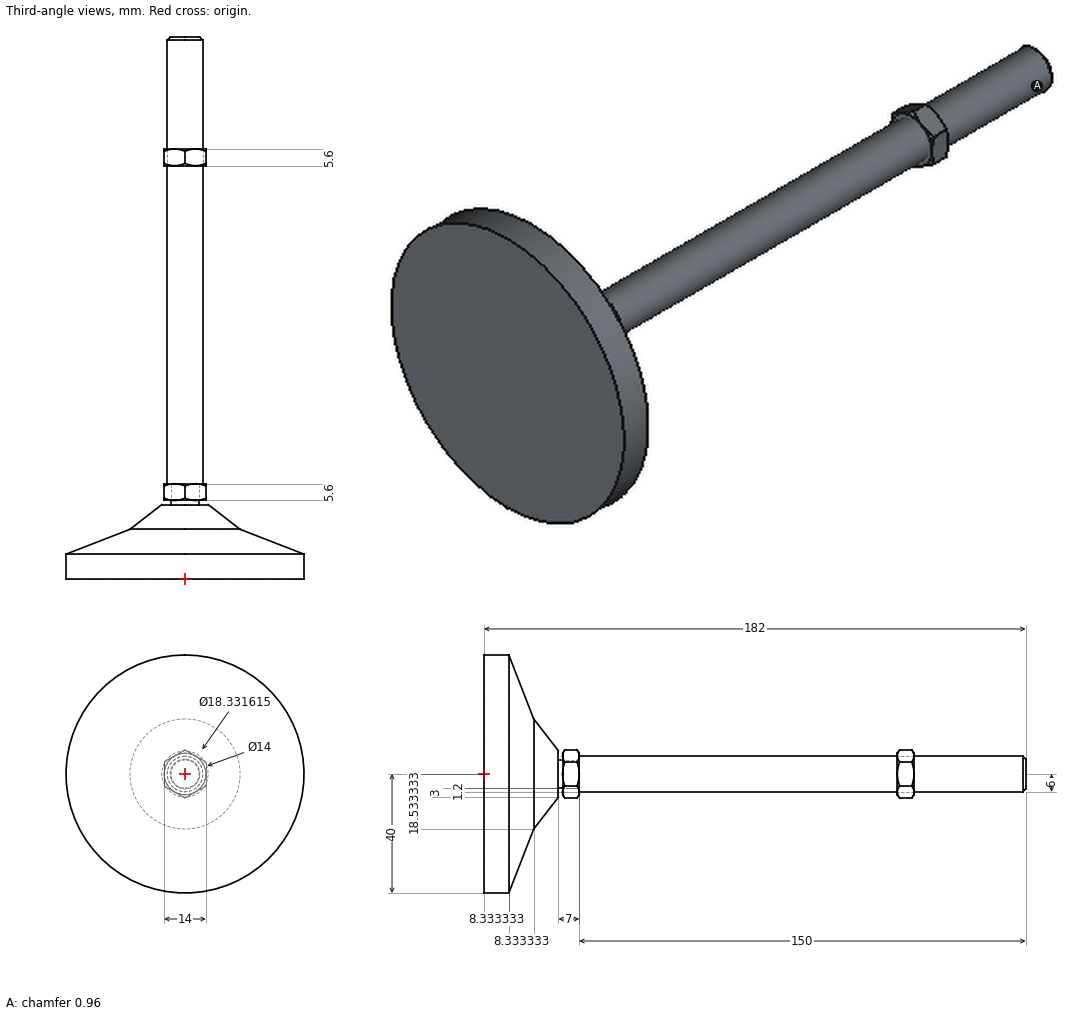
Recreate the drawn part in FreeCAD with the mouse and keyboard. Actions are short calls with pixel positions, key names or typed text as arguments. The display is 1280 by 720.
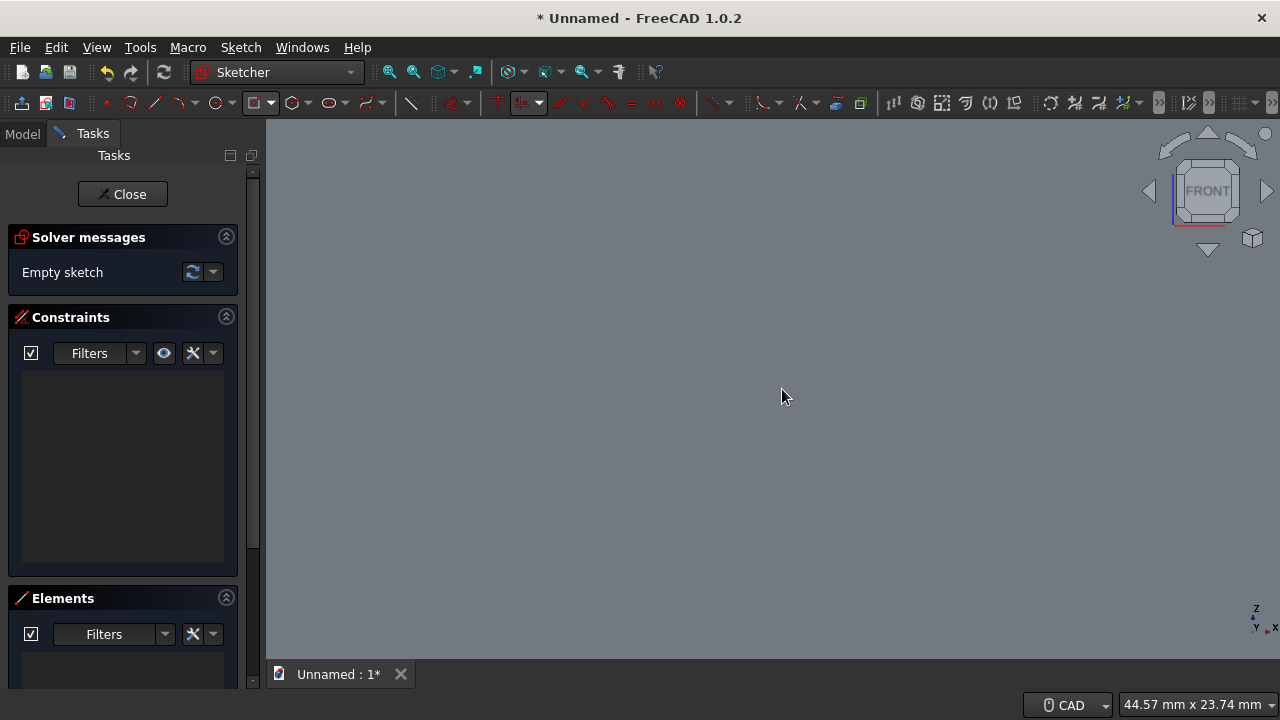
click(292, 104)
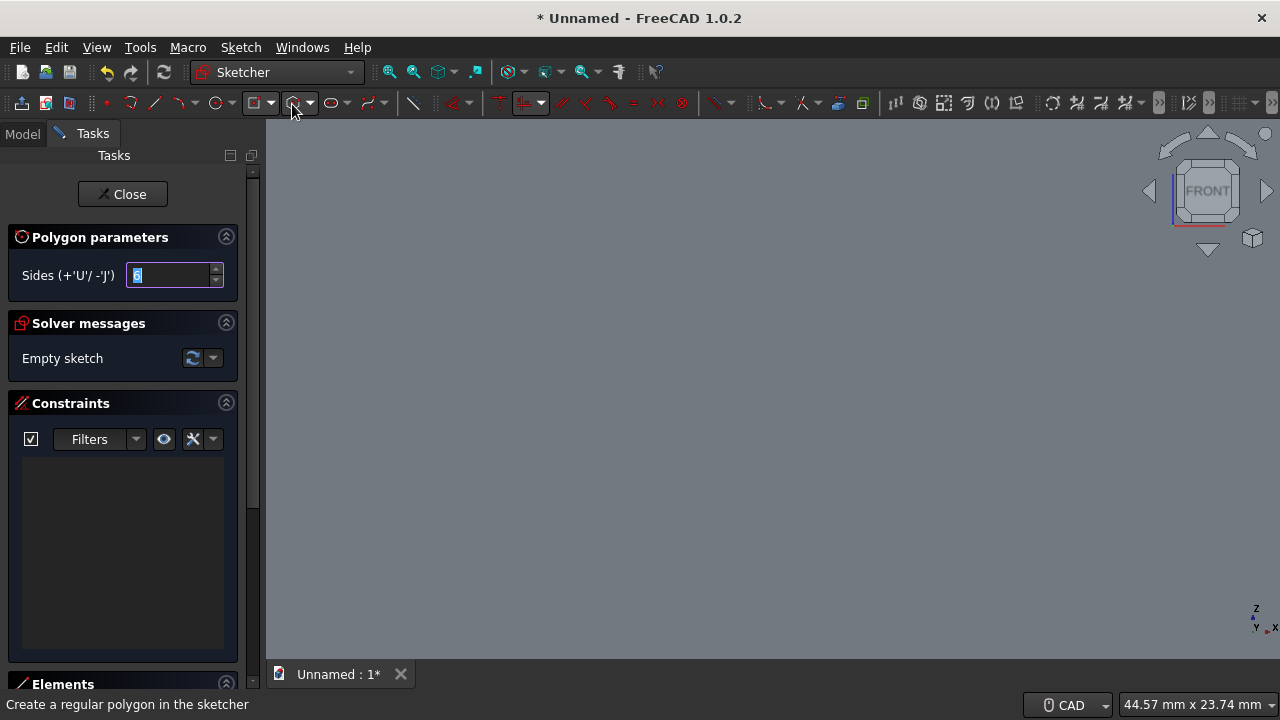
click(697, 385)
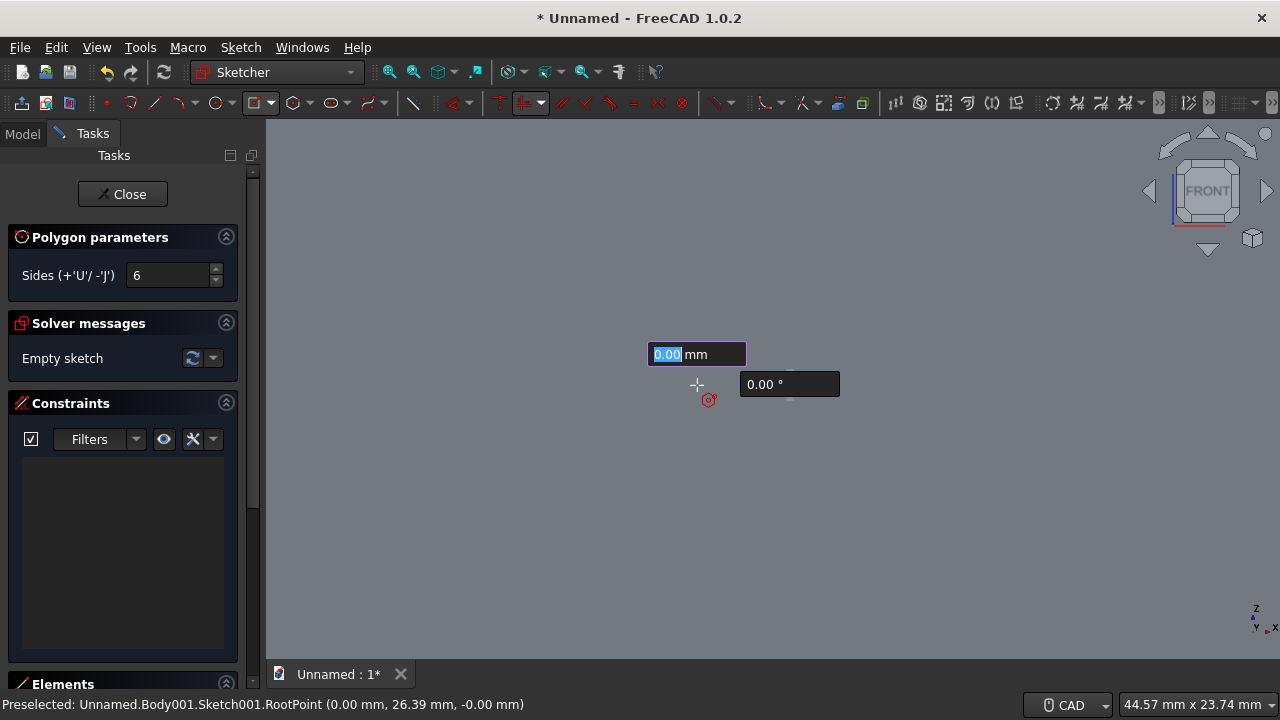
click(697, 569)
right_click(697, 569)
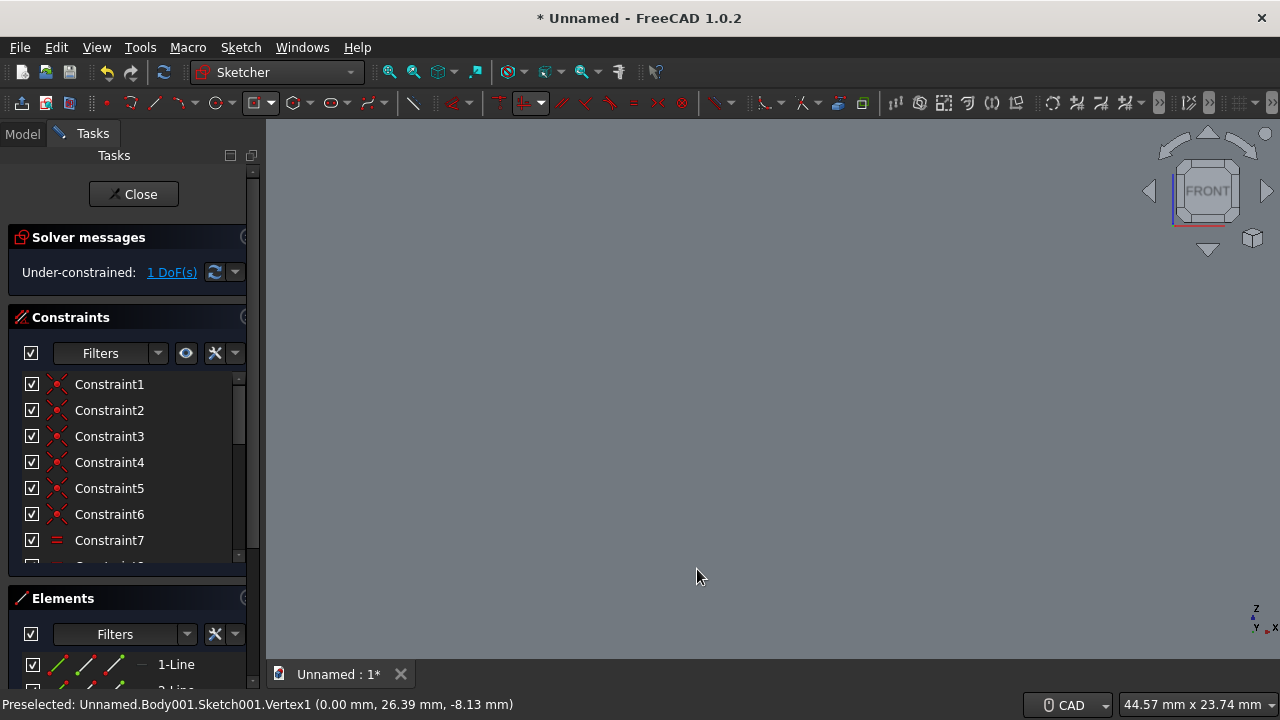
click(452, 104)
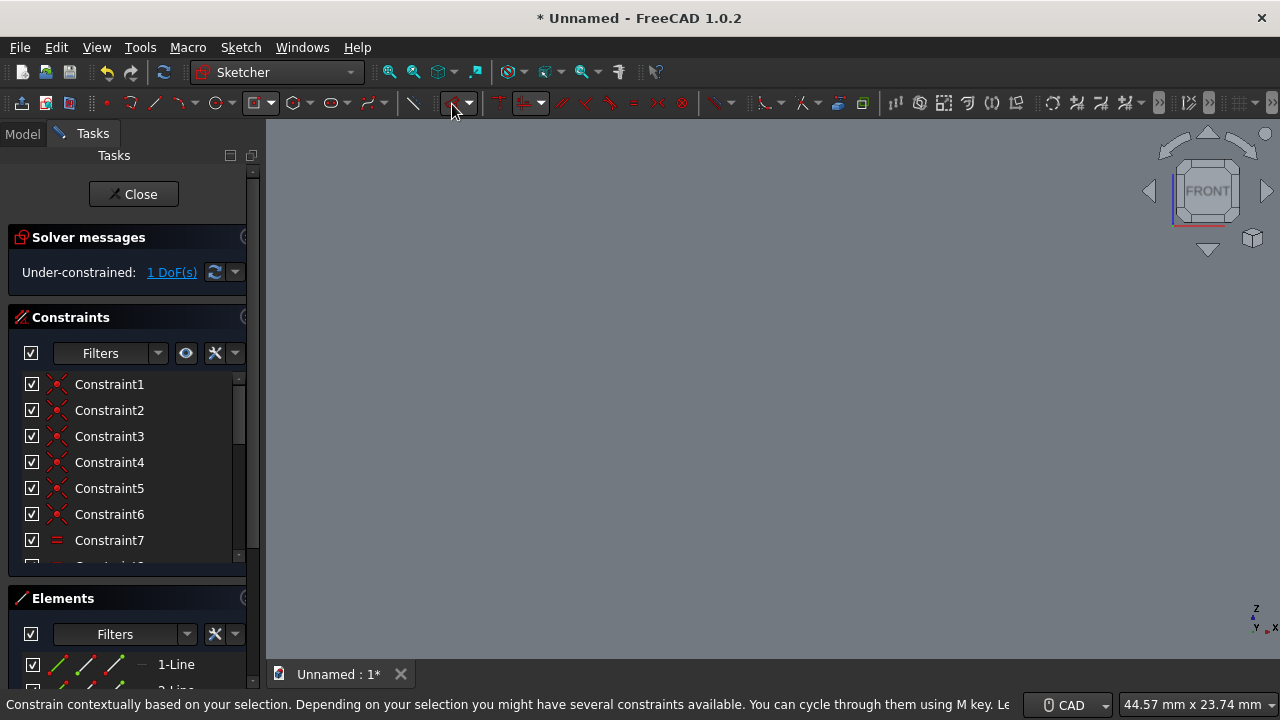
click(536, 292)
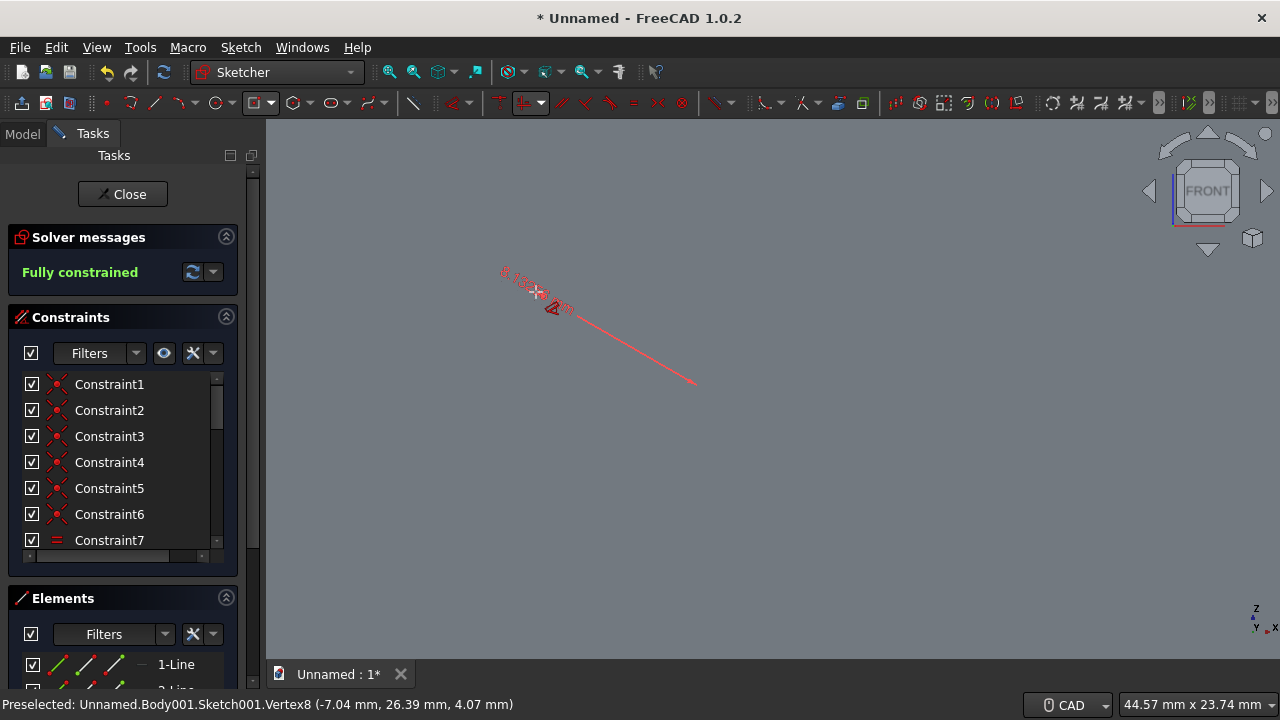
click(857, 477)
click(623, 511)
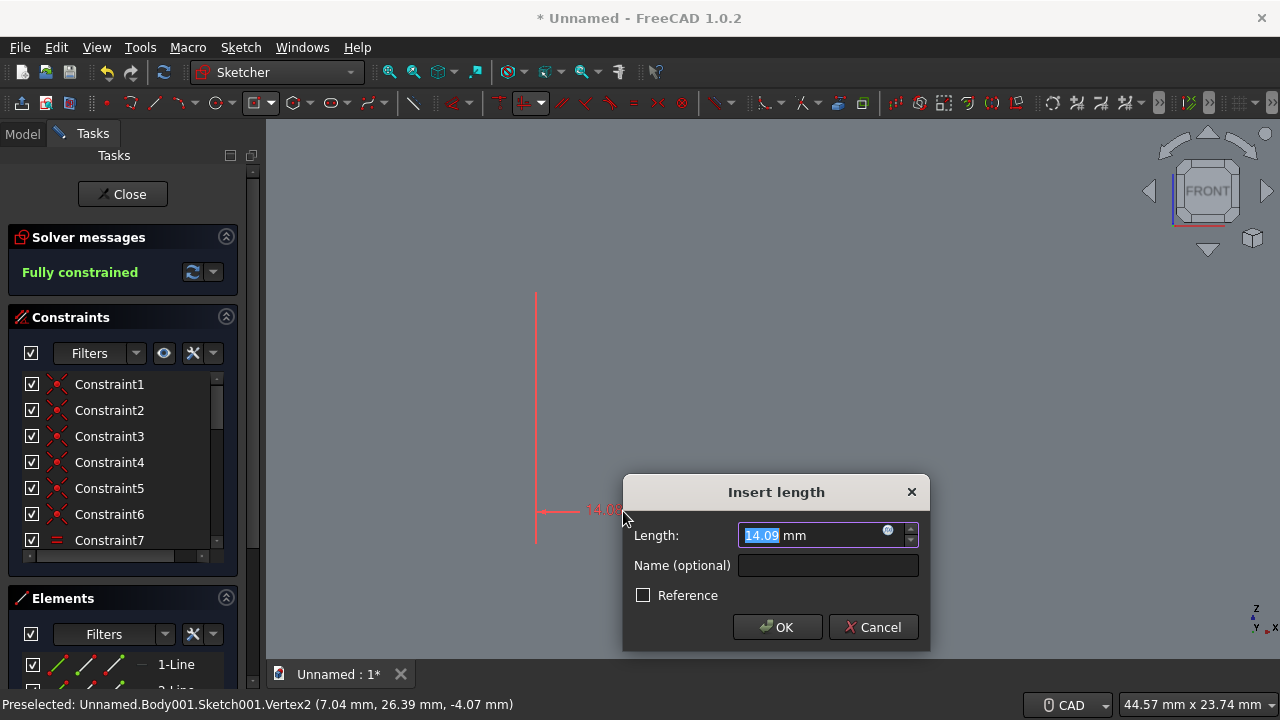
text(14)
key(Return)
key(Escape)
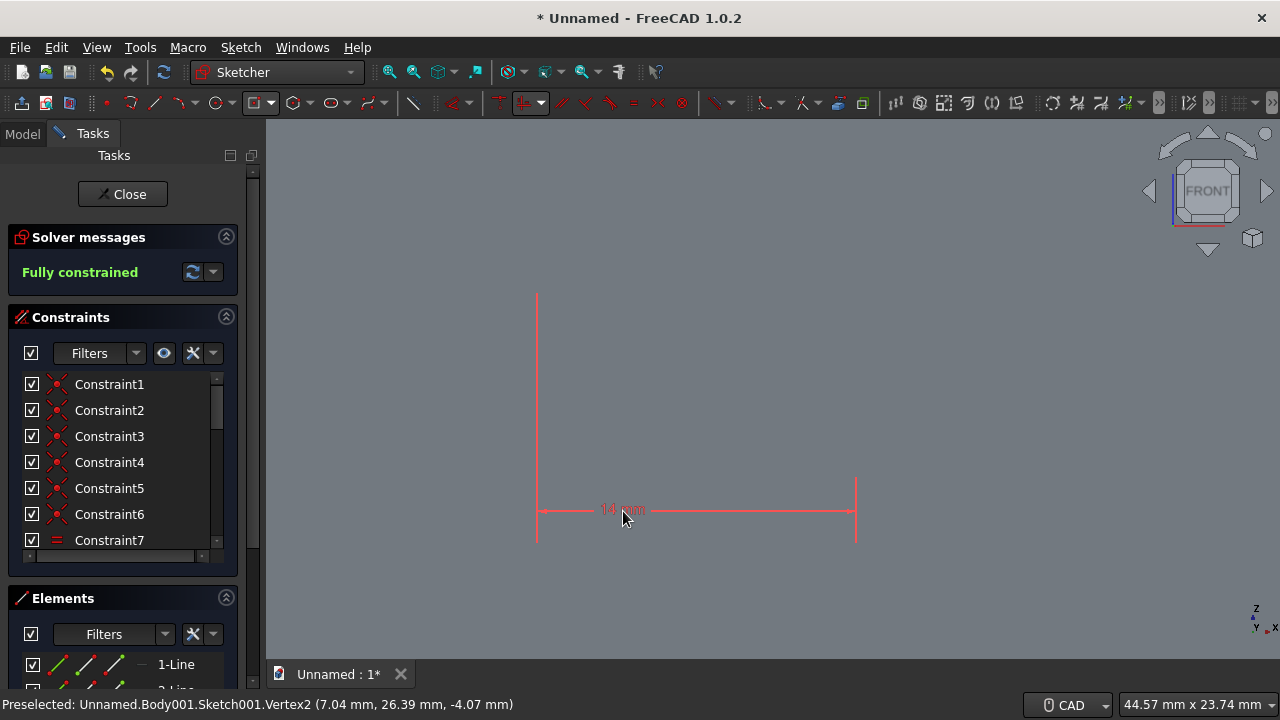
click(123, 194)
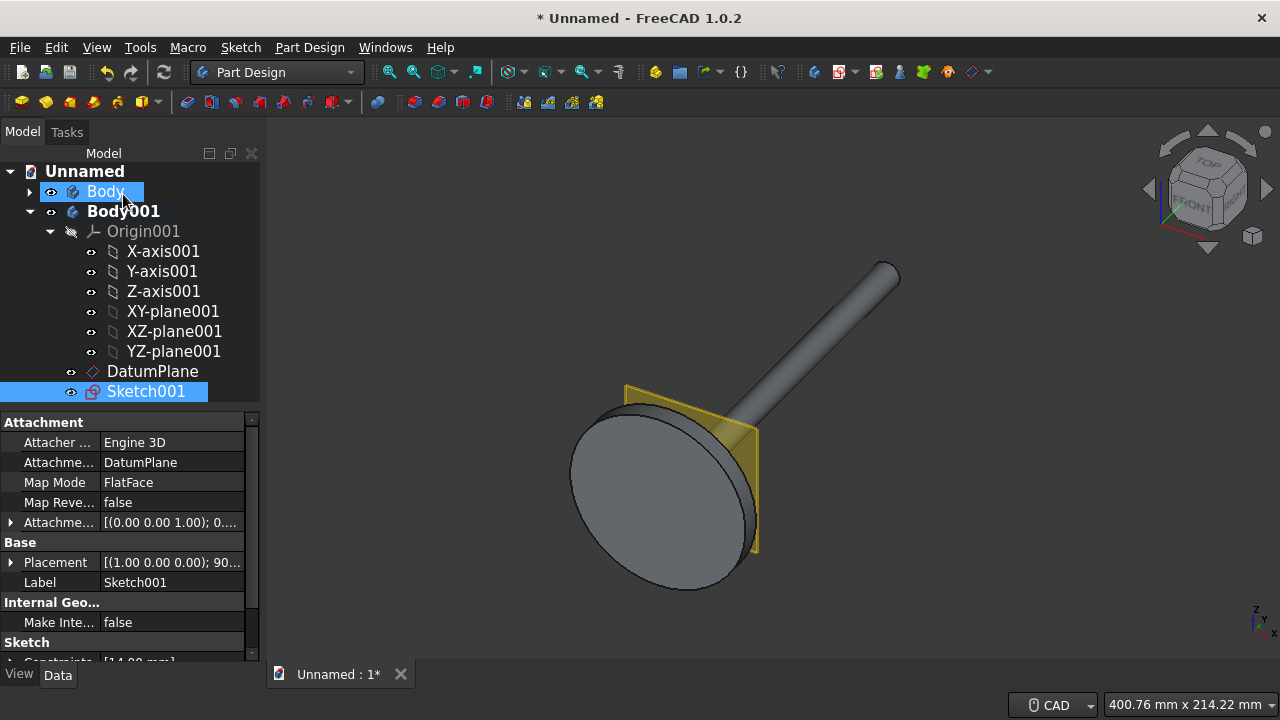
click(22, 102)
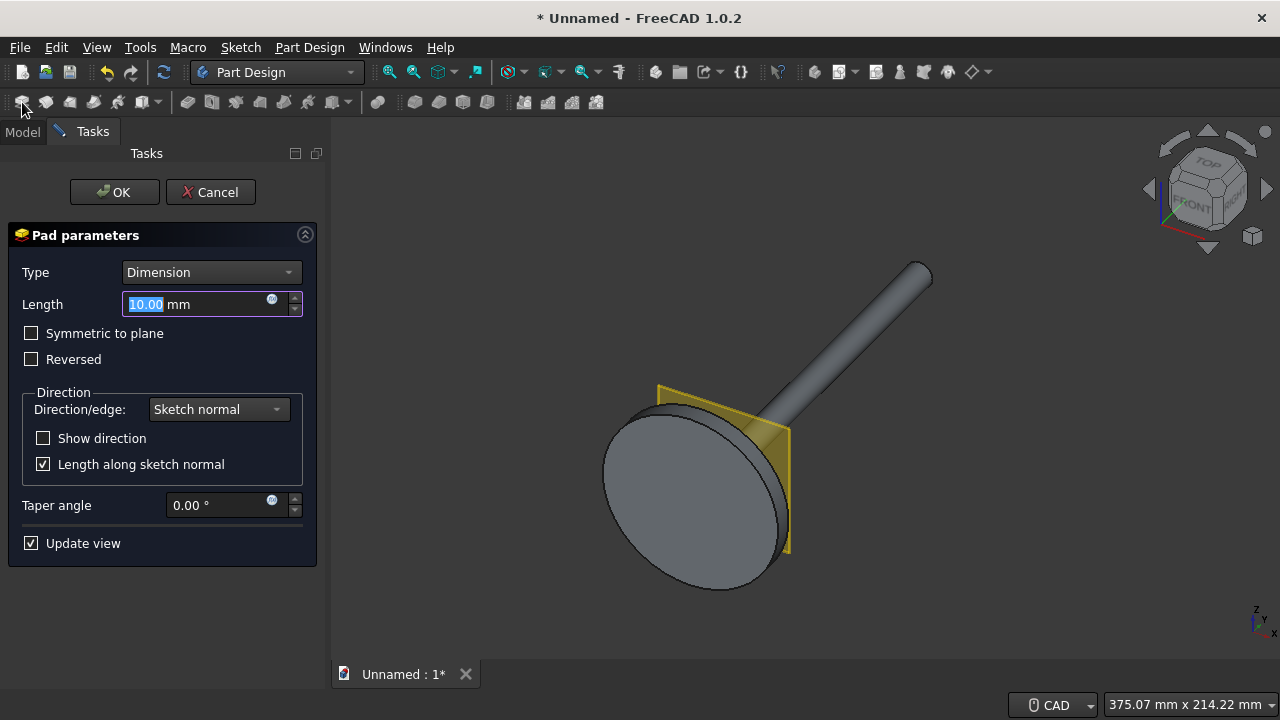
text(5.6)
key(Tab)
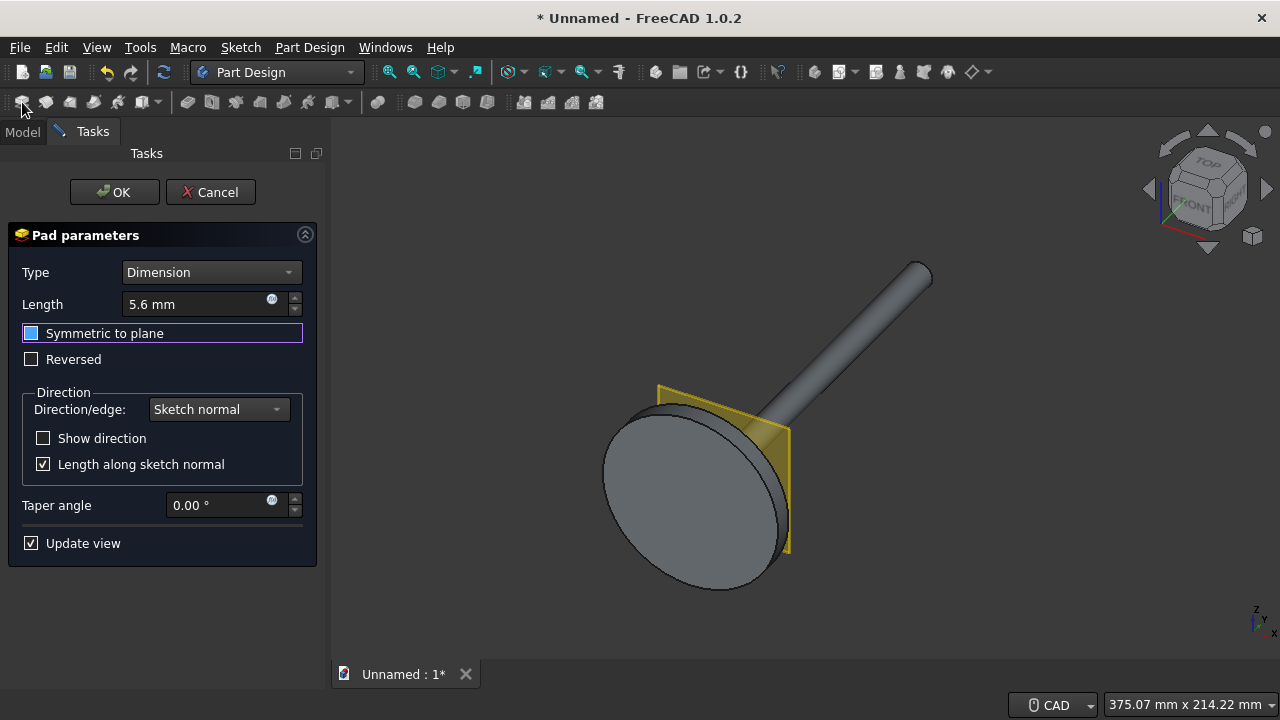
click(30, 359)